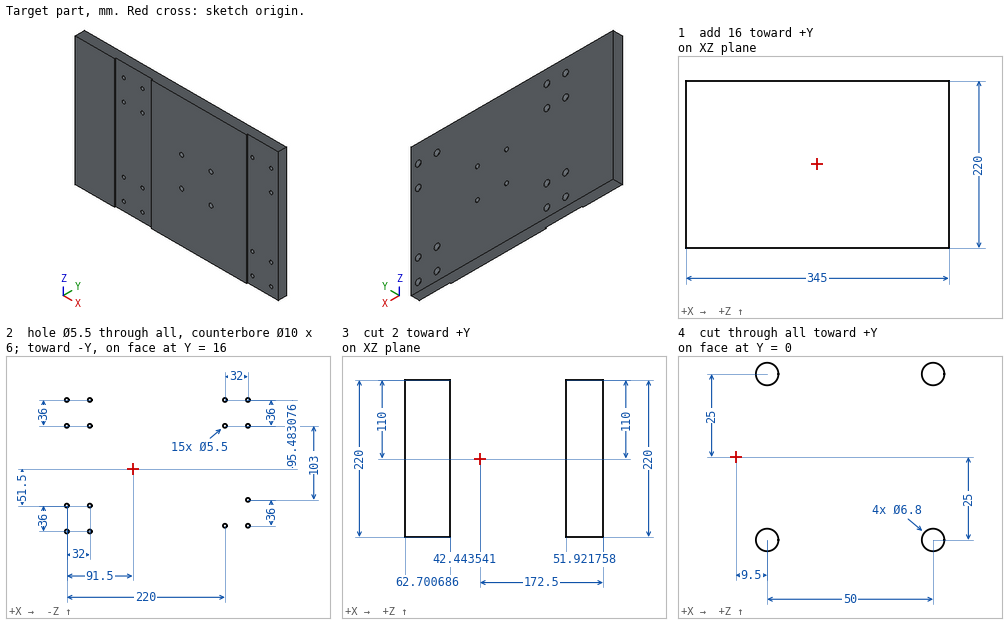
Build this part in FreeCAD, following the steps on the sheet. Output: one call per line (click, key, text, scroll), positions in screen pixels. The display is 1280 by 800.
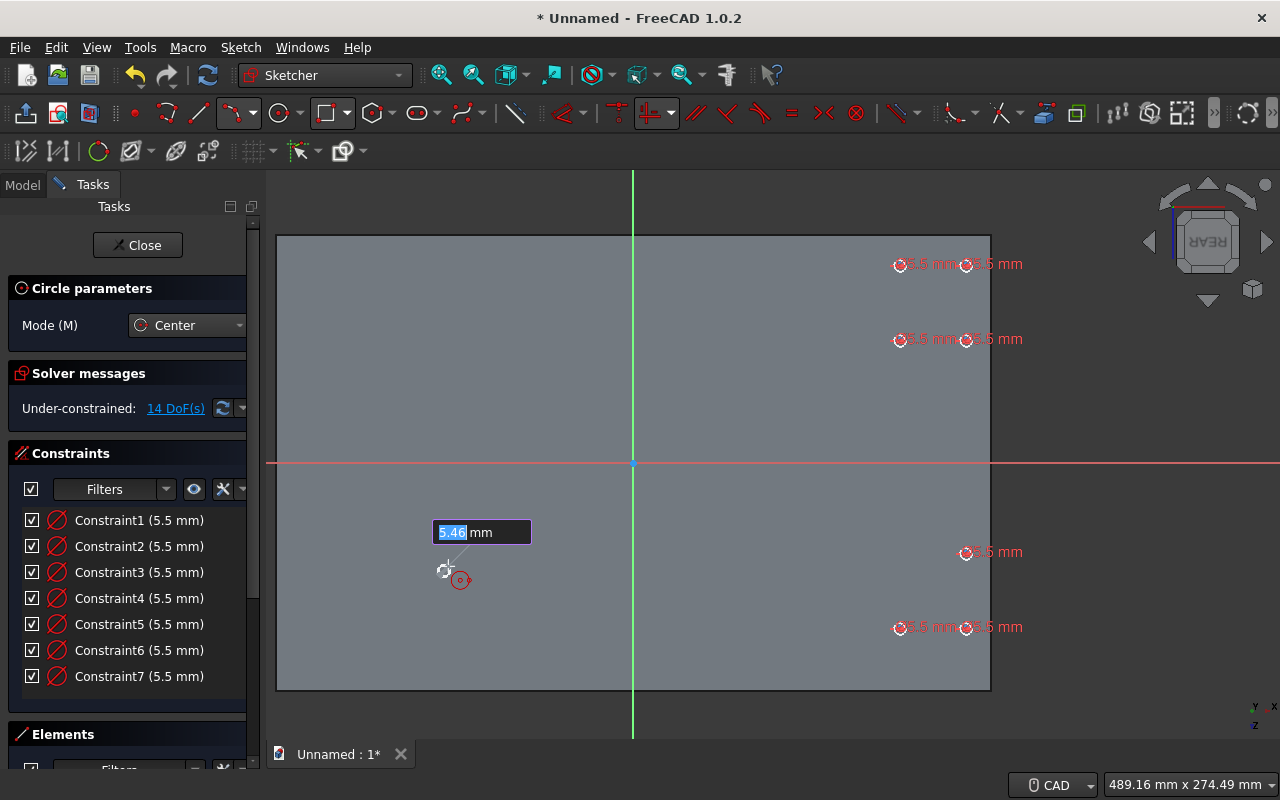
text(5.5)
key(Return)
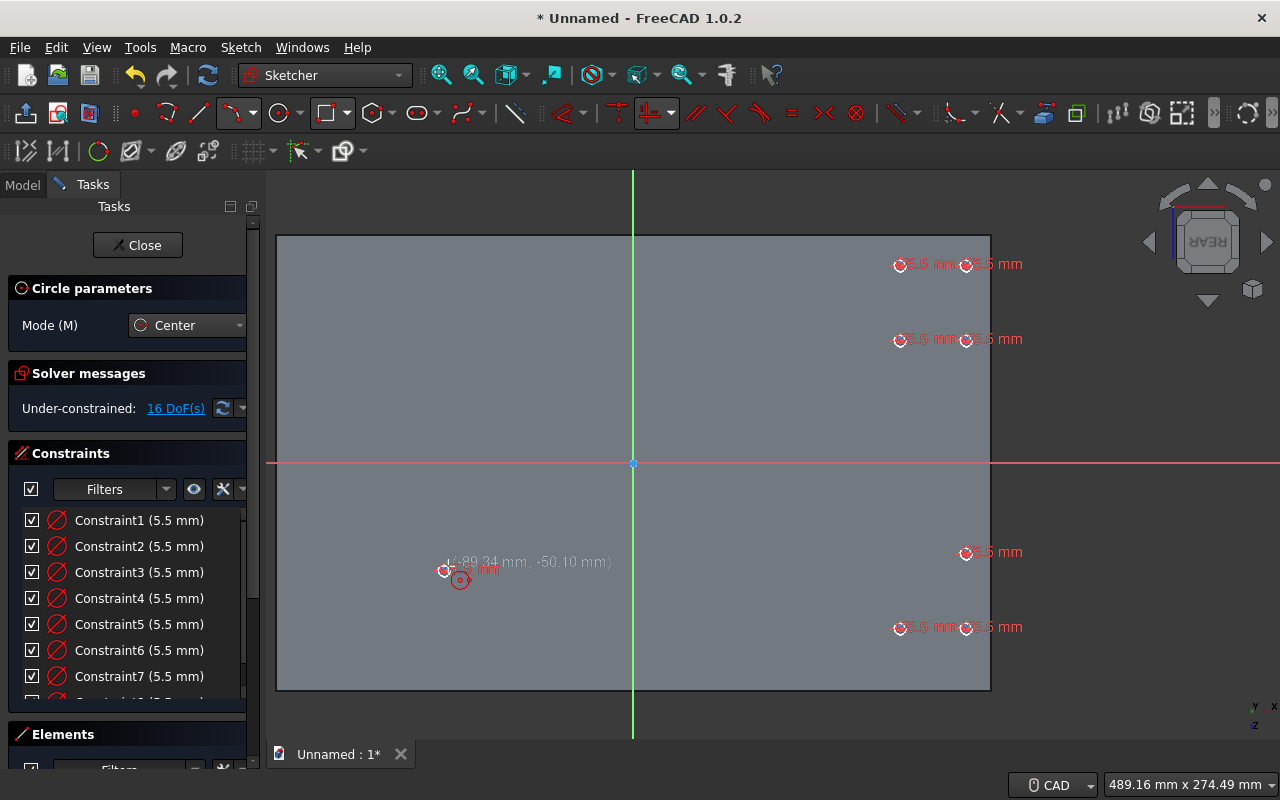
scroll(510, 570, up, 7)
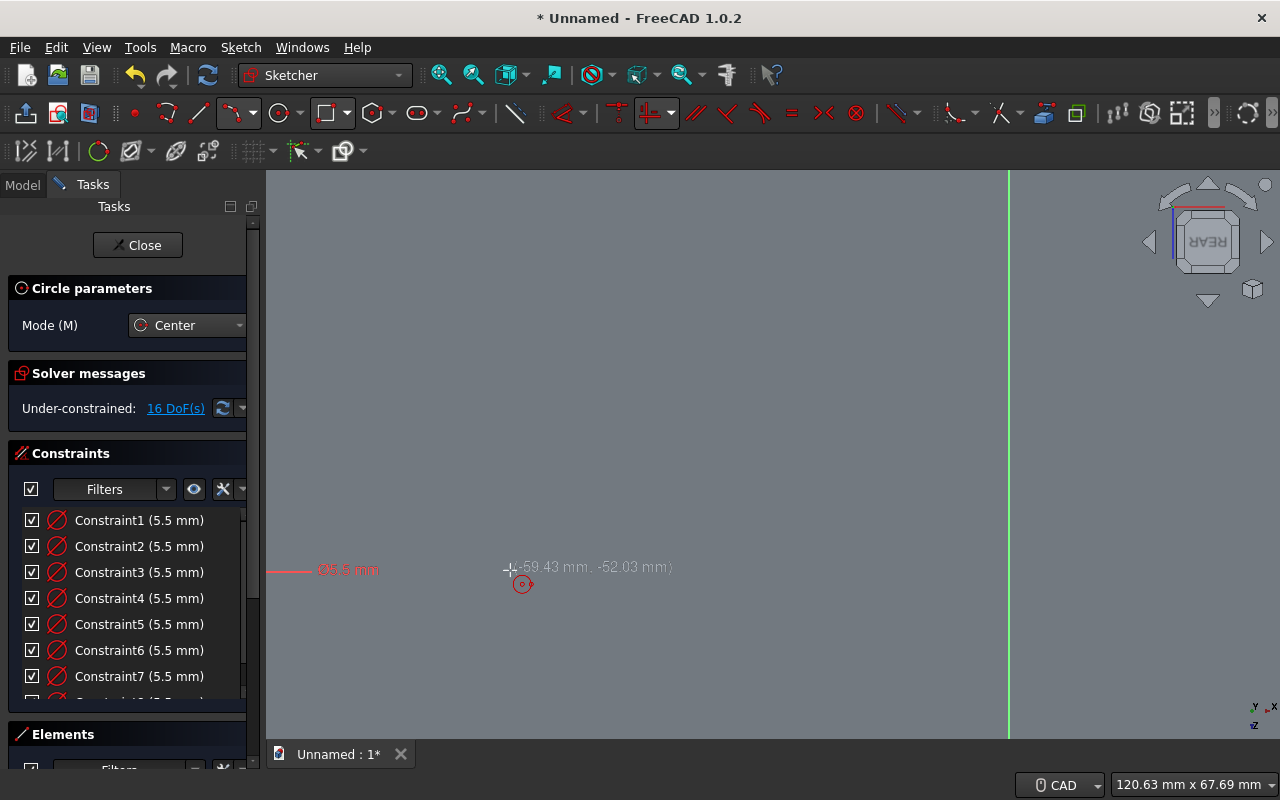
scroll(510, 570, down, 7)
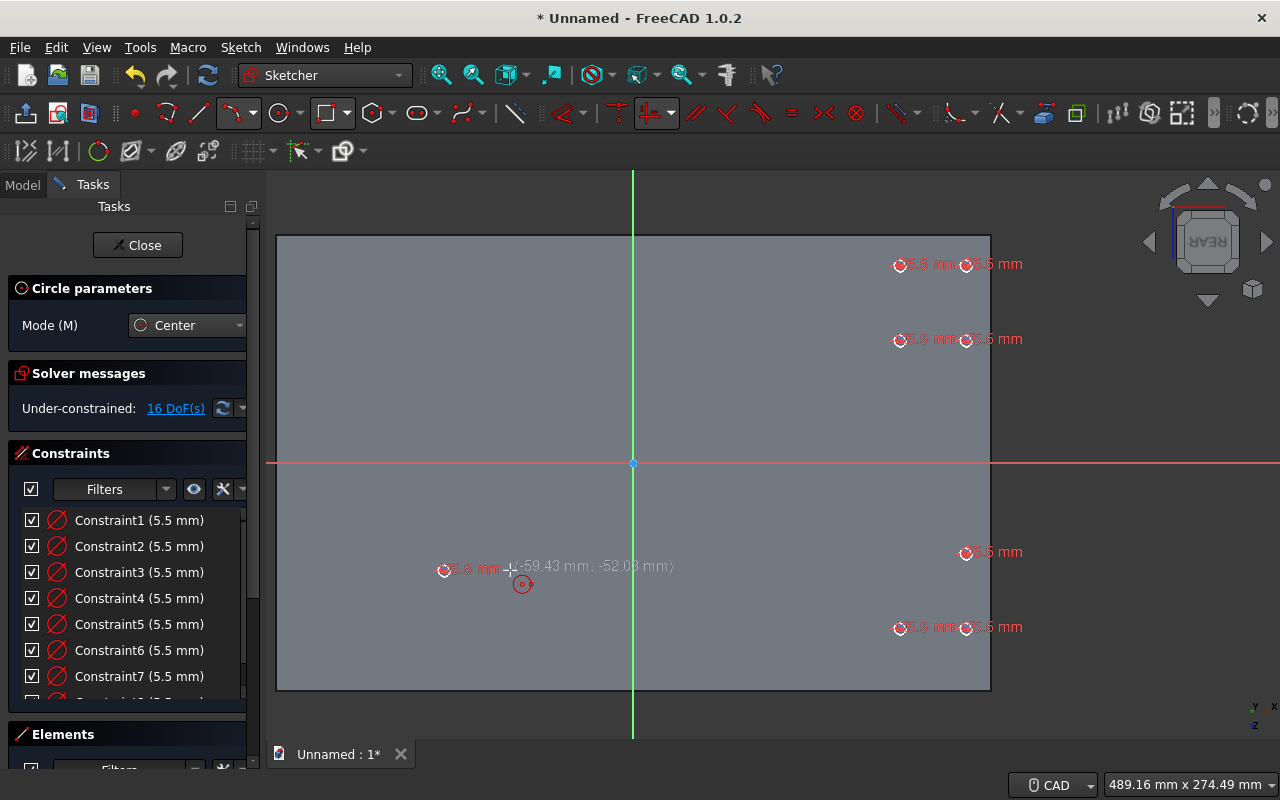
click(510, 570)
move(514, 566)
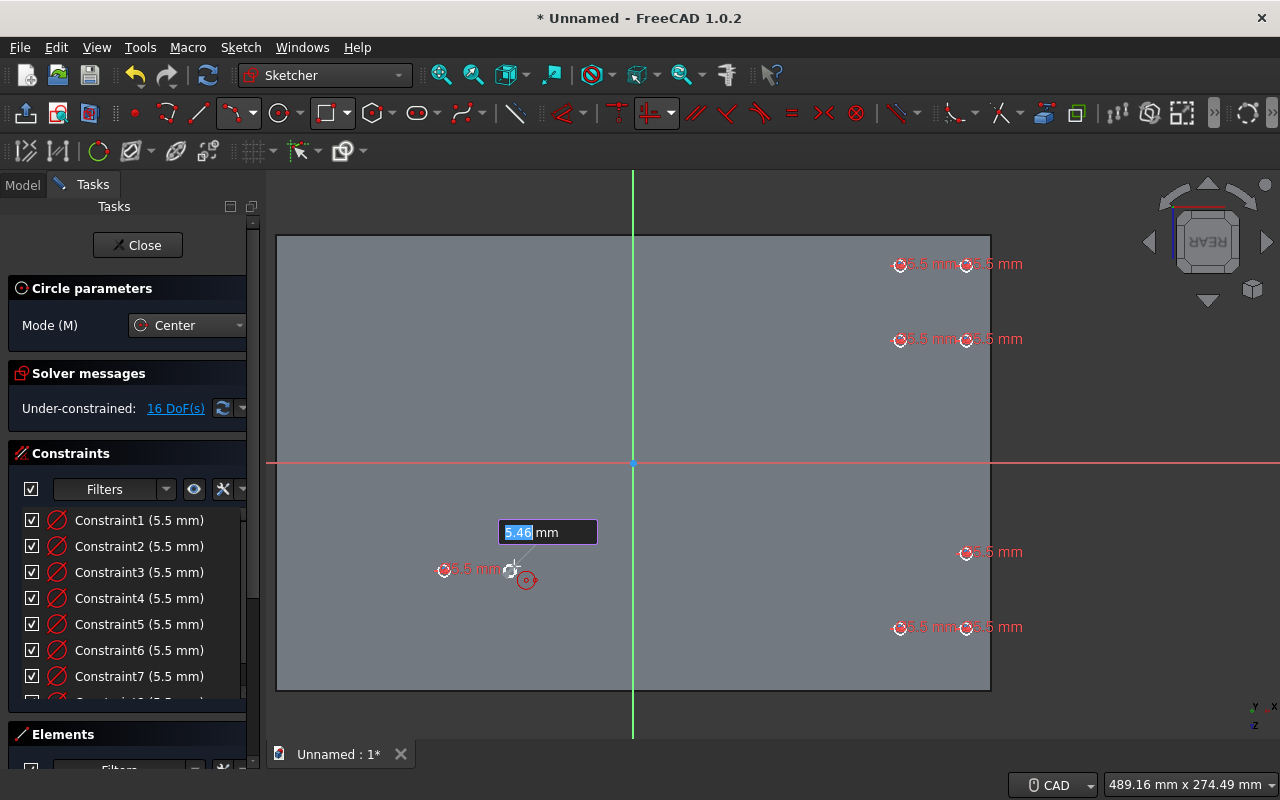
text(5.5)
key(Return)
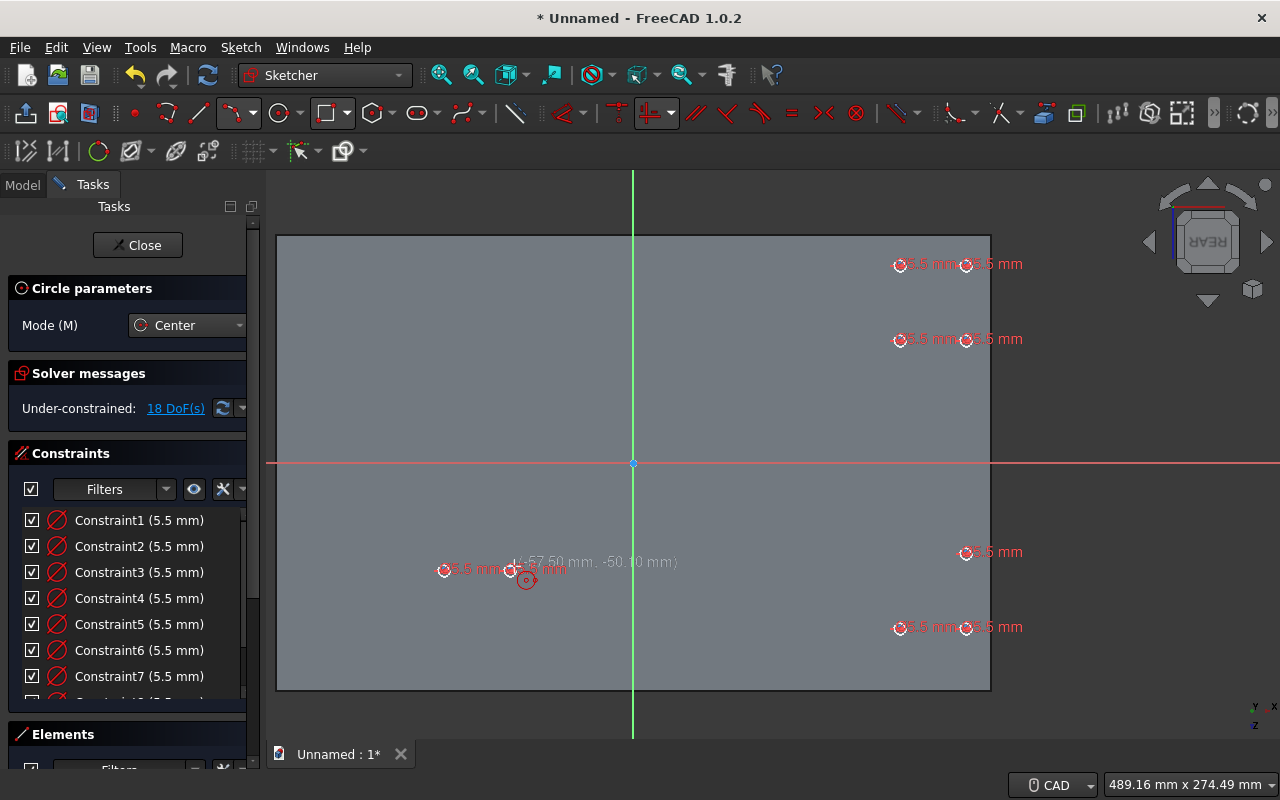
scroll(510, 645, up, 7)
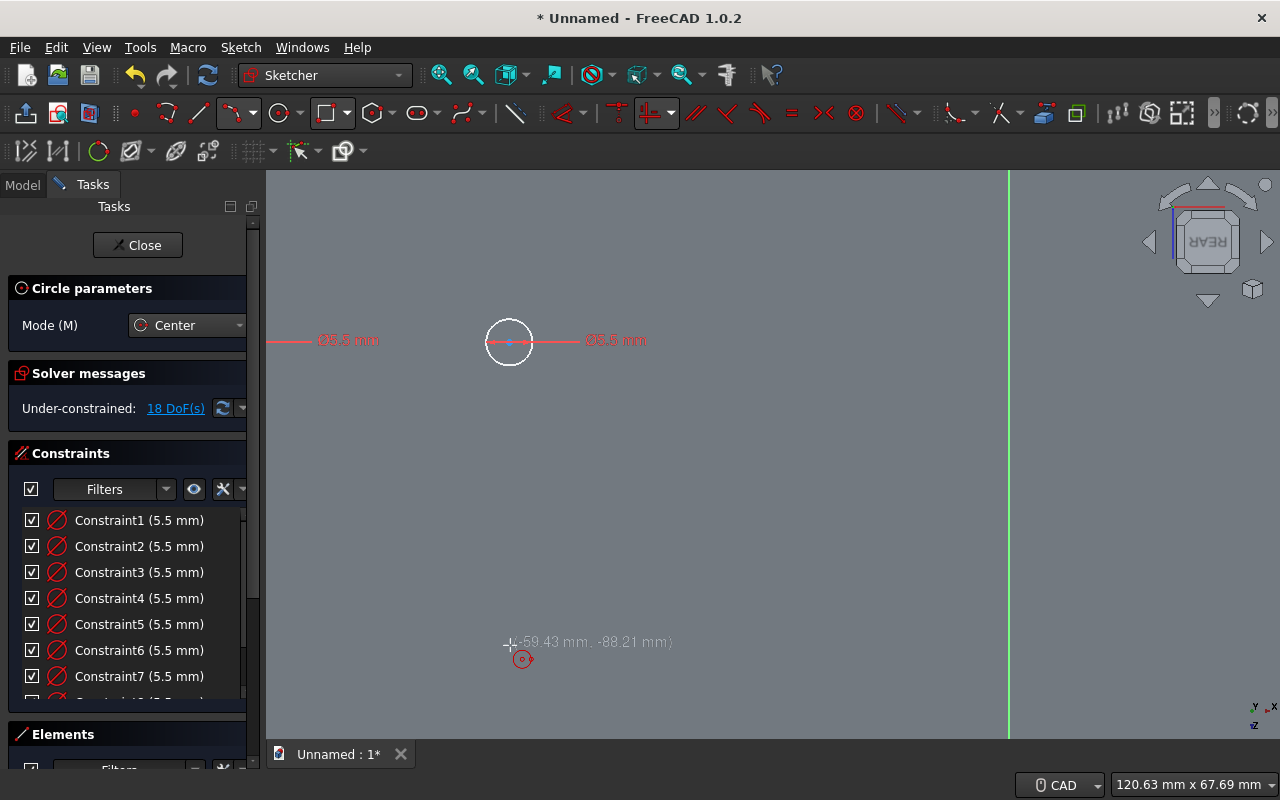
scroll(510, 645, down, 7)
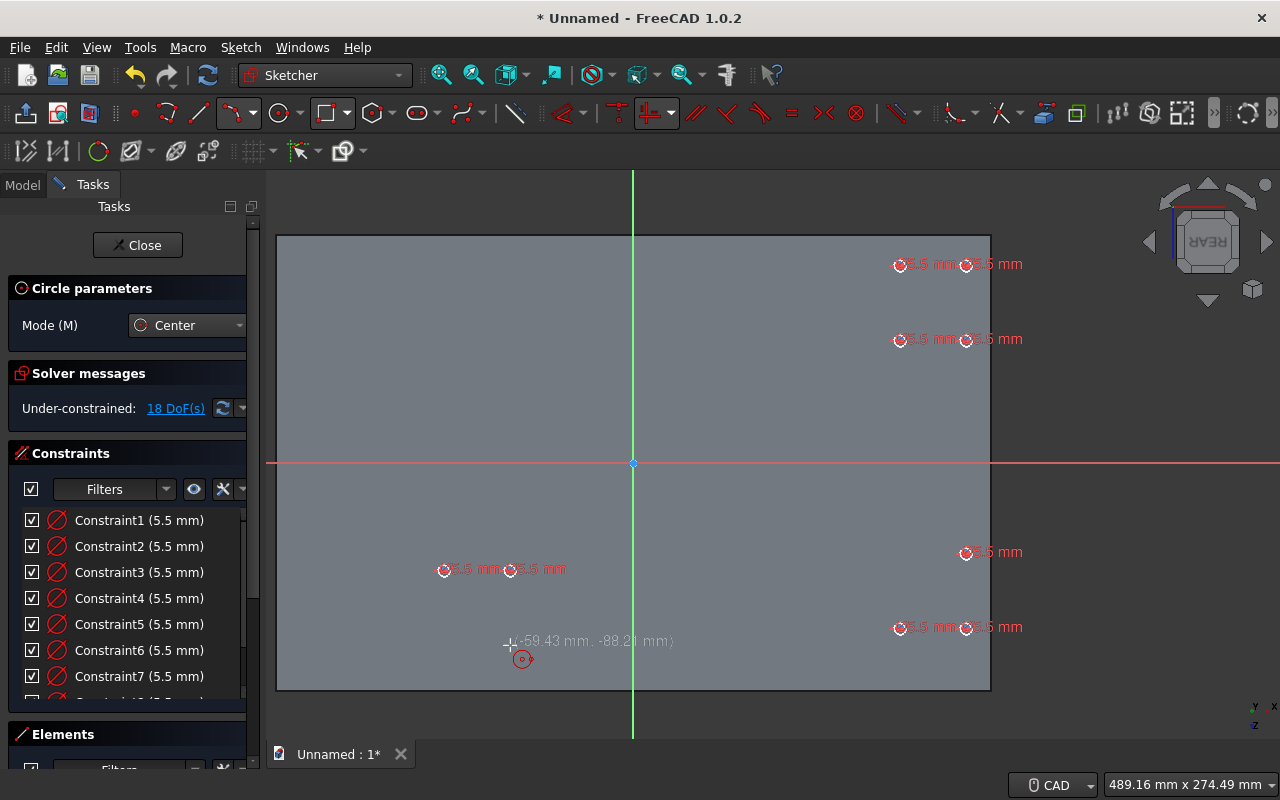
click(510, 645)
move(514, 640)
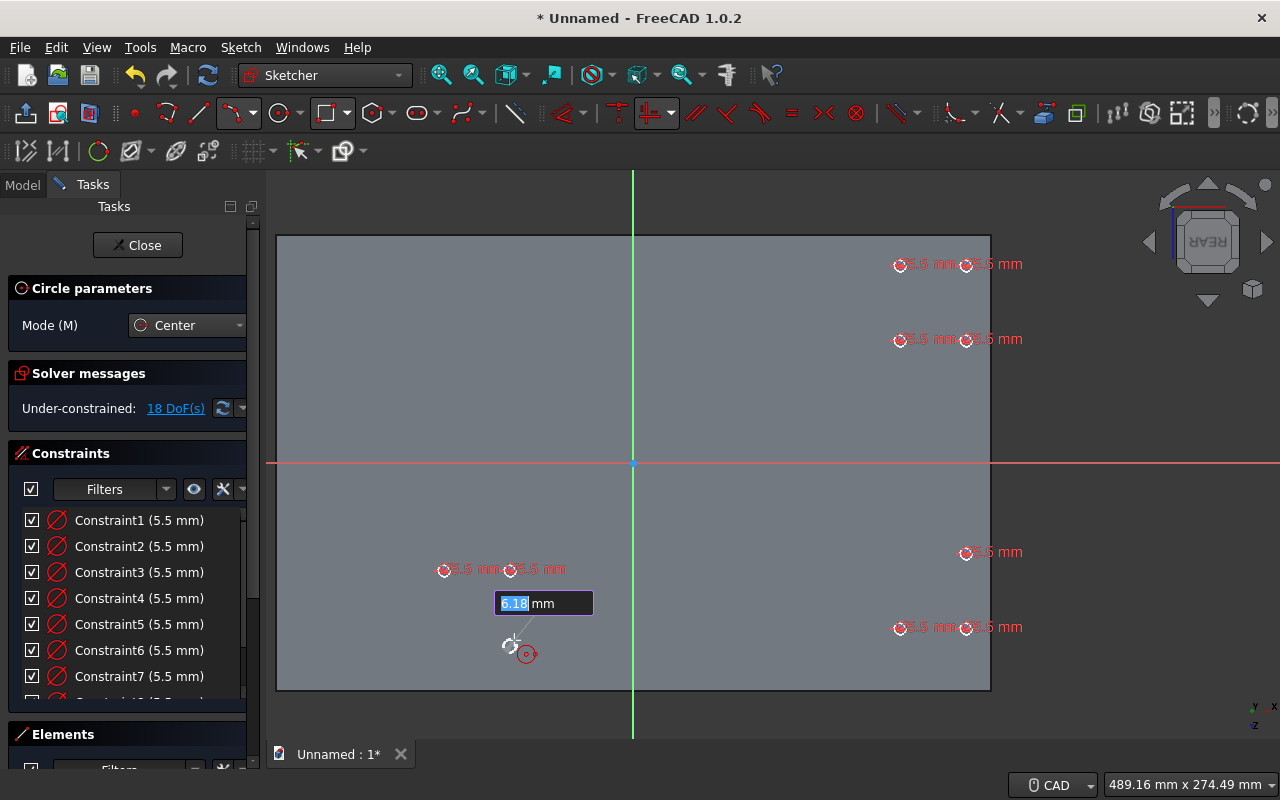
text(5.5)
key(Return)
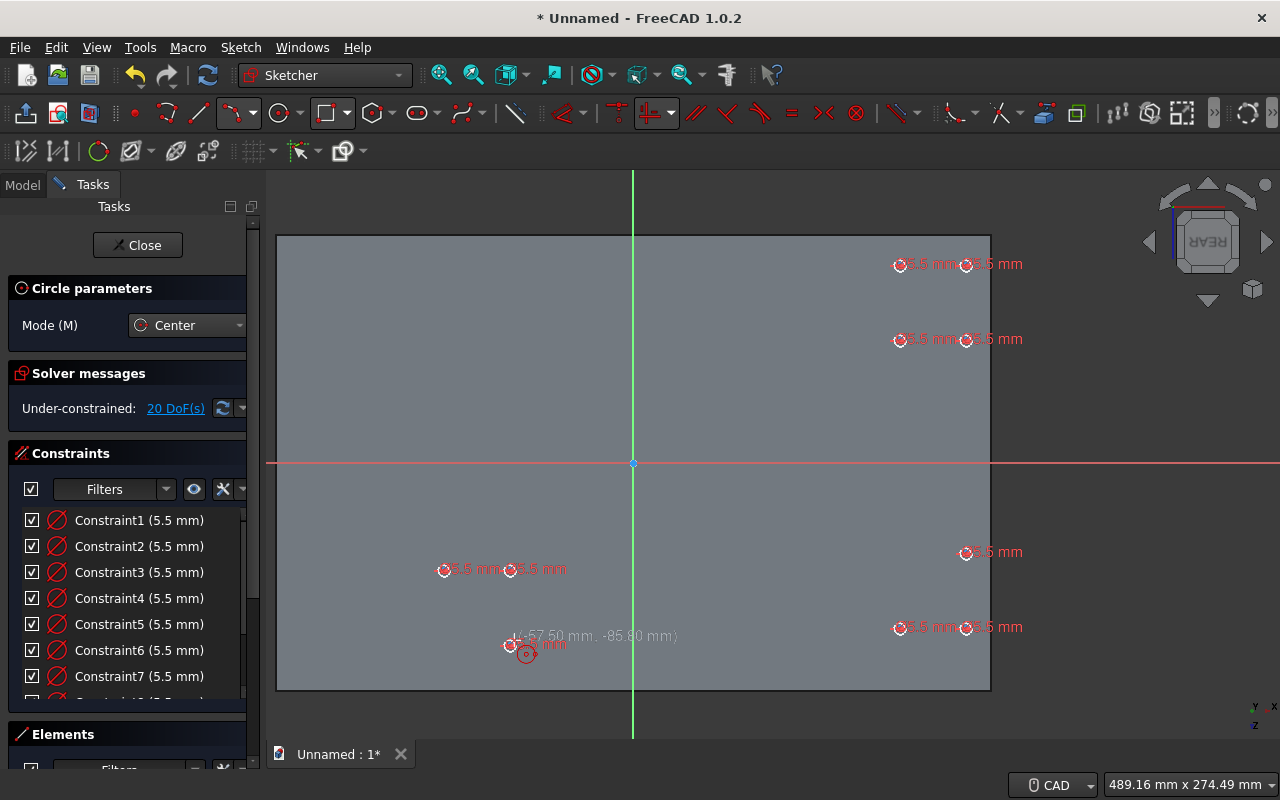
scroll(444, 645, up, 7)